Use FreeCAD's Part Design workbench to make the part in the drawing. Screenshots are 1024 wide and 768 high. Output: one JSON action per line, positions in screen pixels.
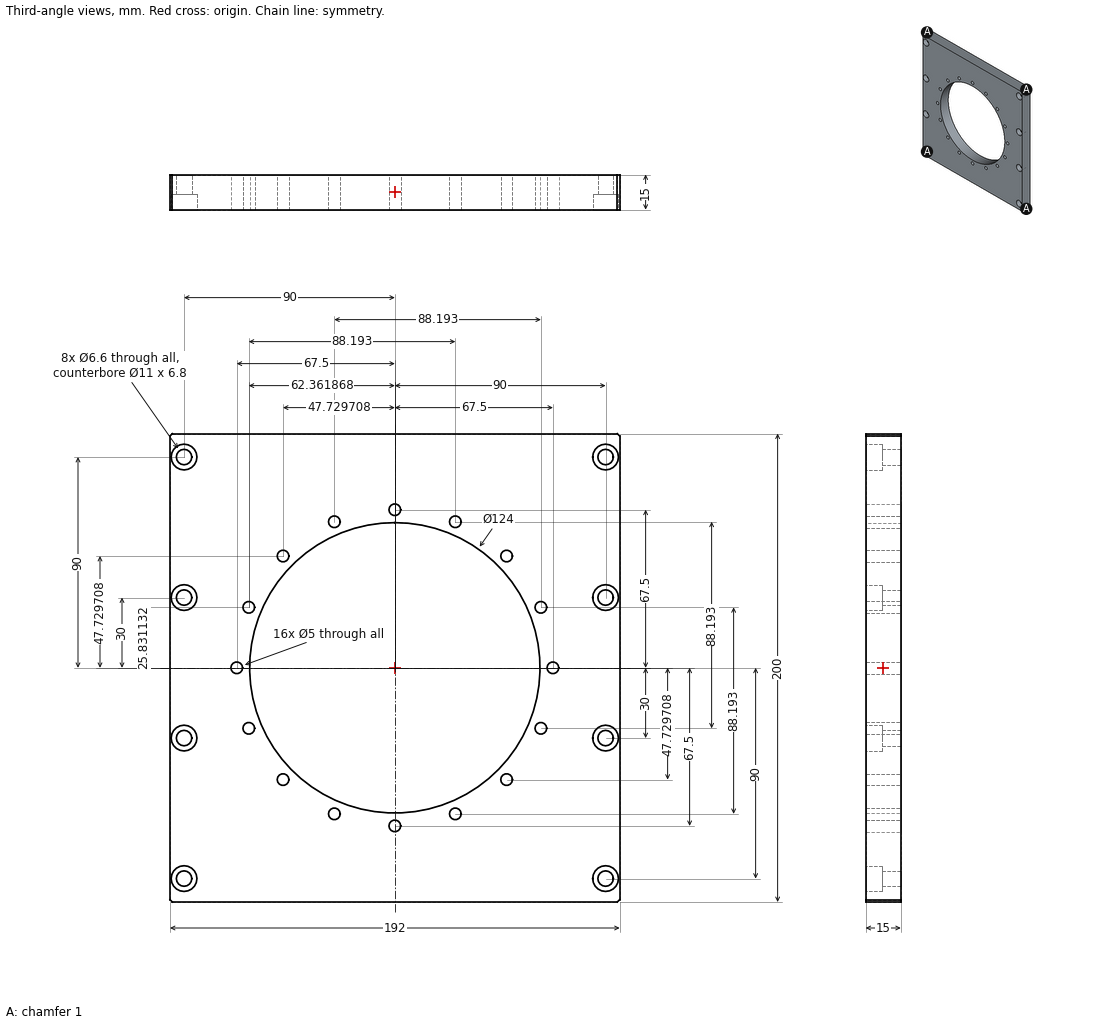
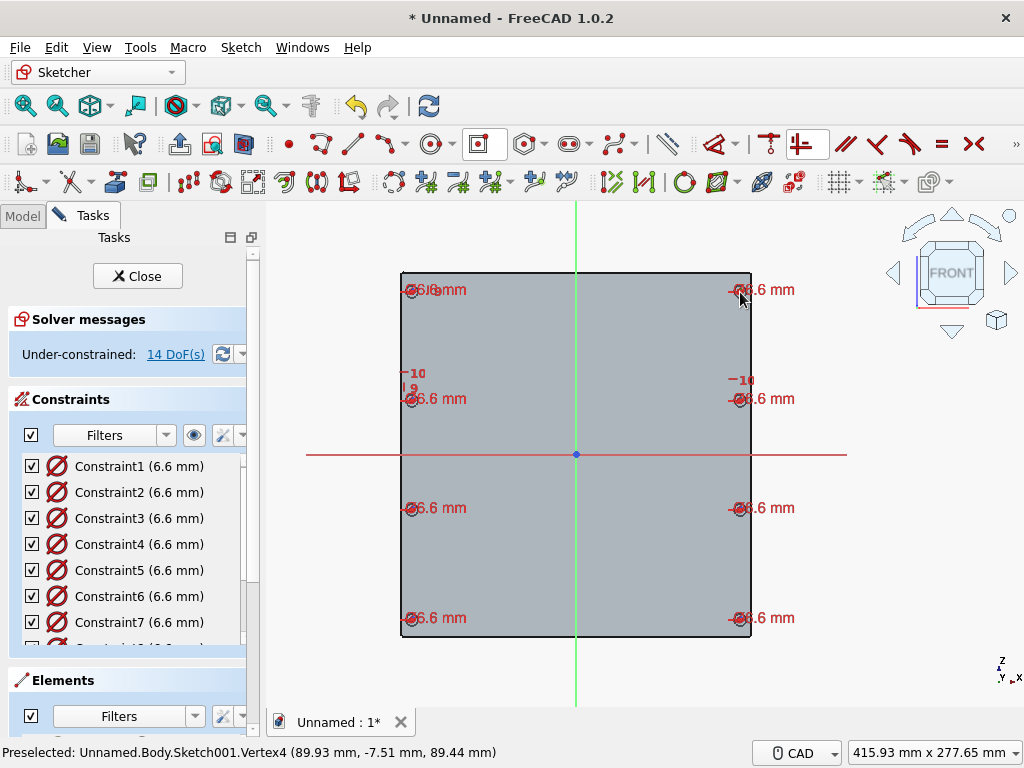
{"action": "left_click", "coordinate": [824, 144]}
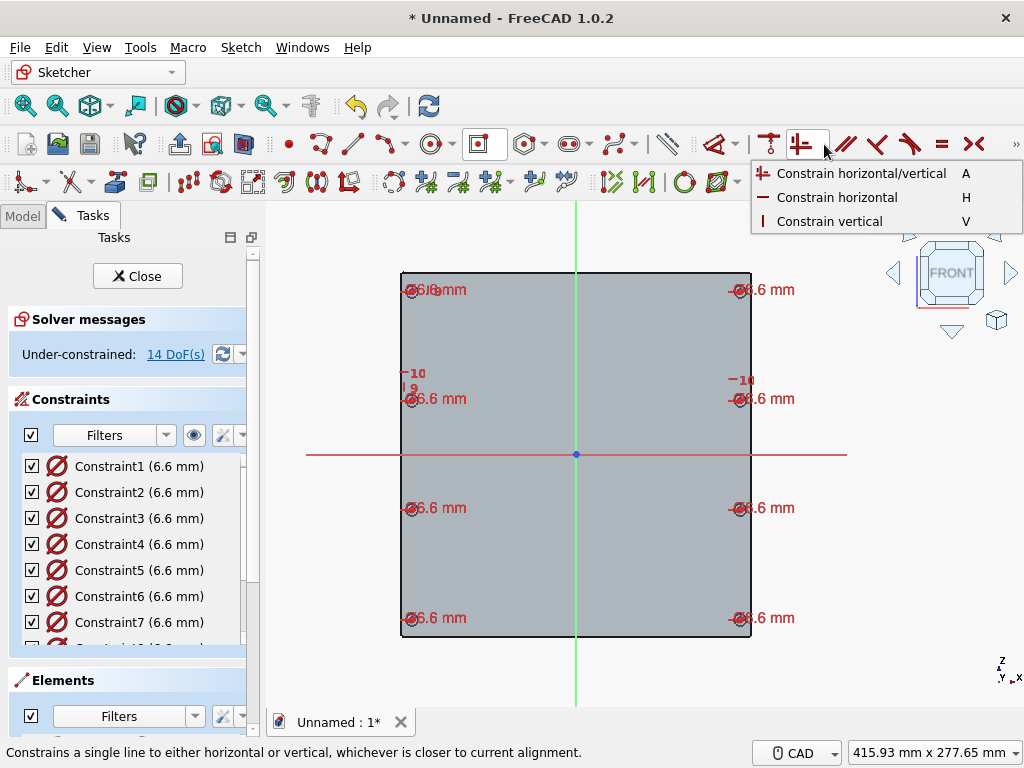
{"action": "left_click", "coordinate": [887, 221]}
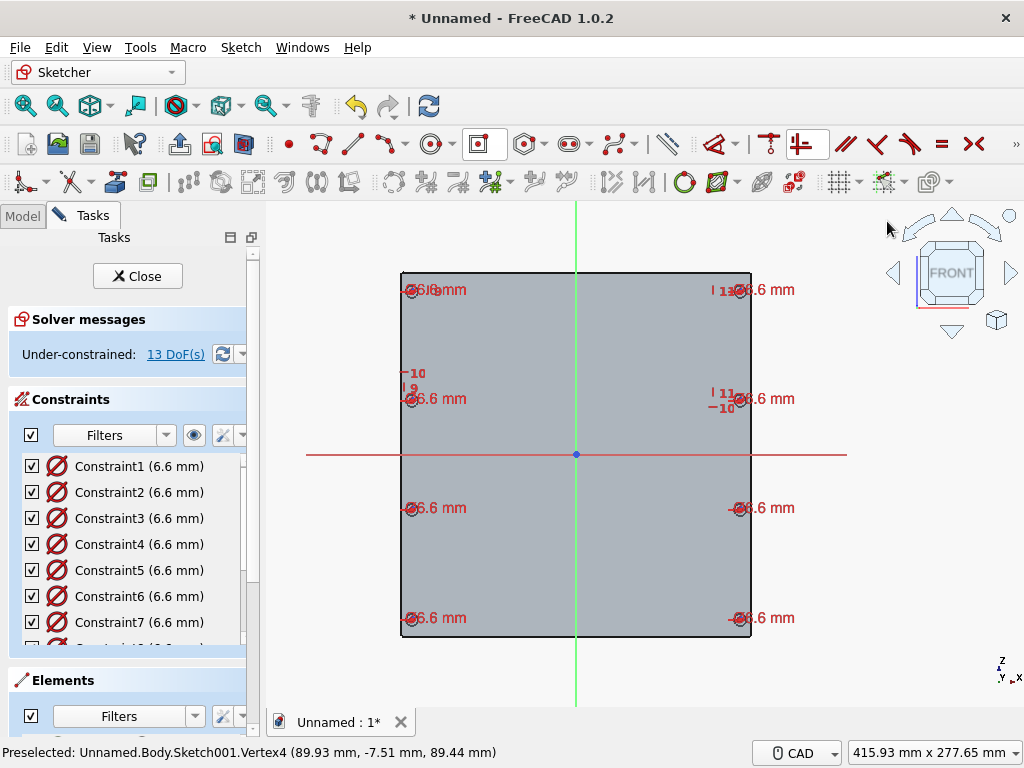
{"action": "left_click", "coordinate": [412, 292]}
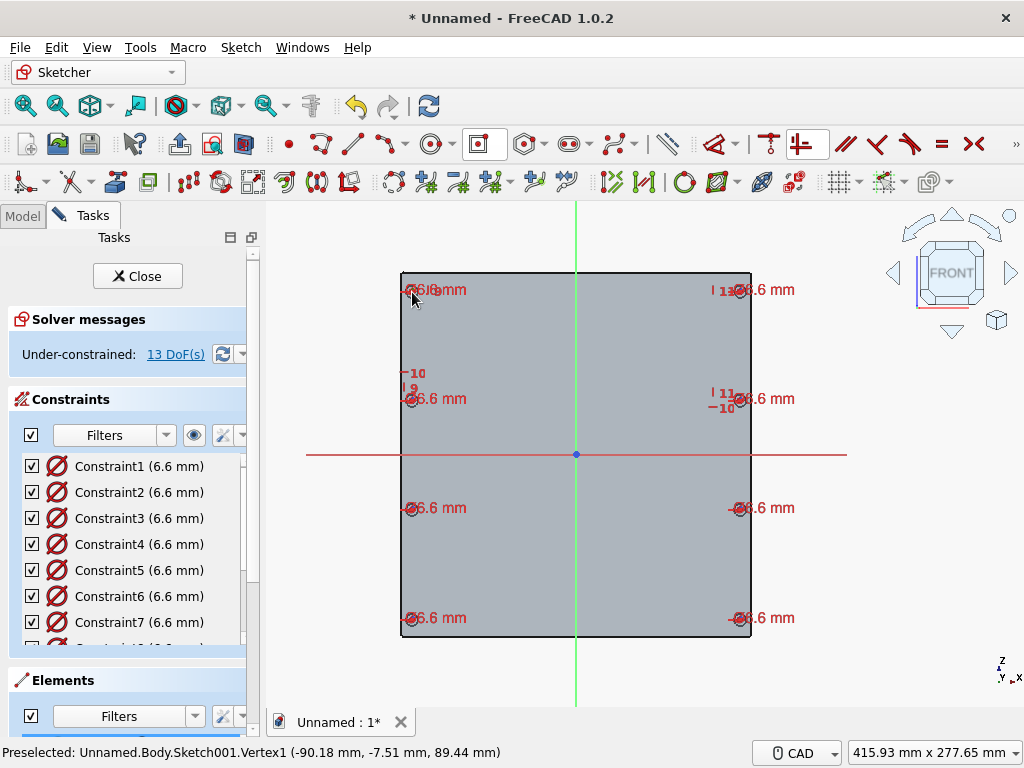
{"action": "left_click", "coordinate": [740, 292]}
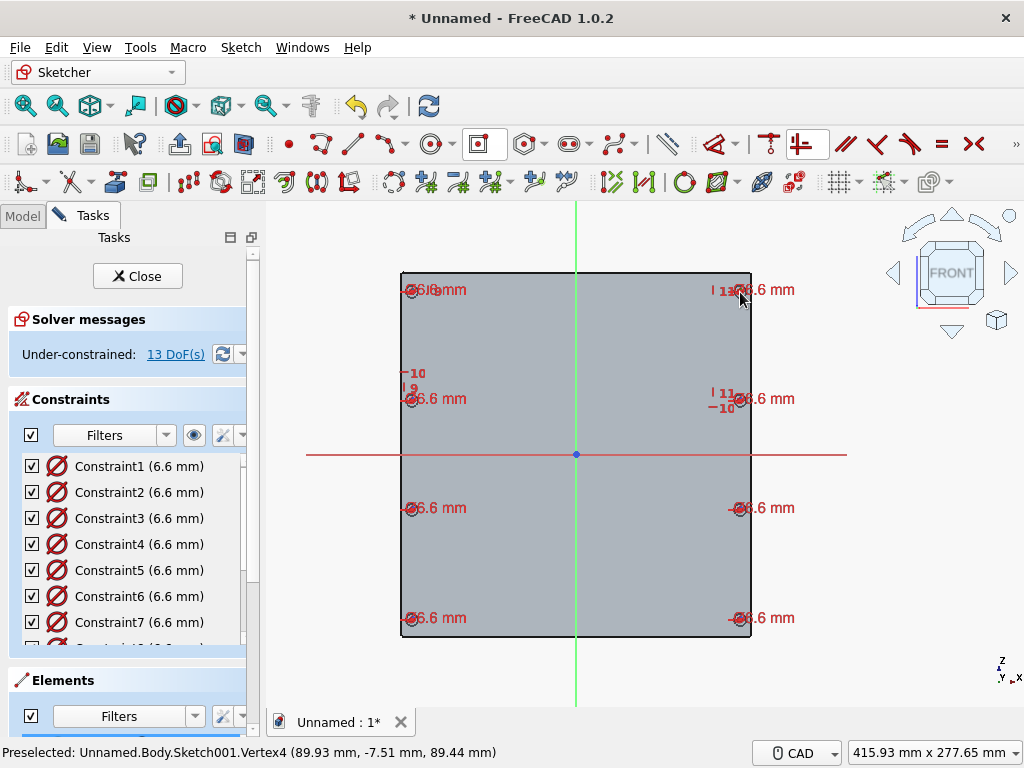
{"action": "left_click", "coordinate": [824, 144]}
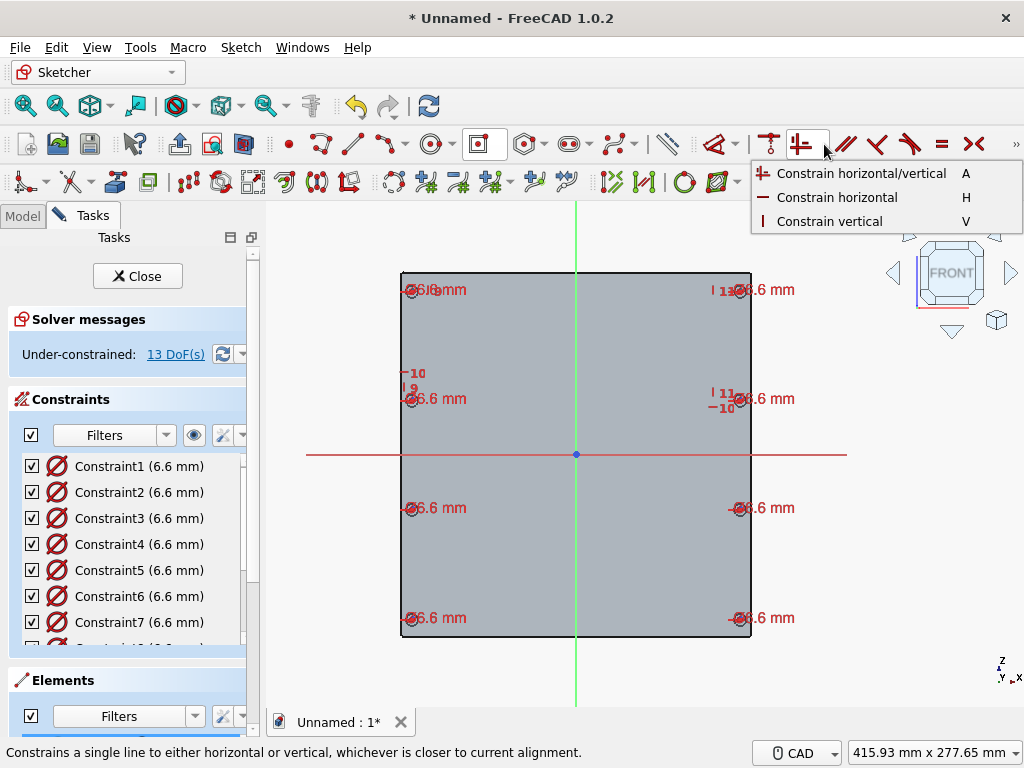
{"action": "left_click", "coordinate": [887, 197]}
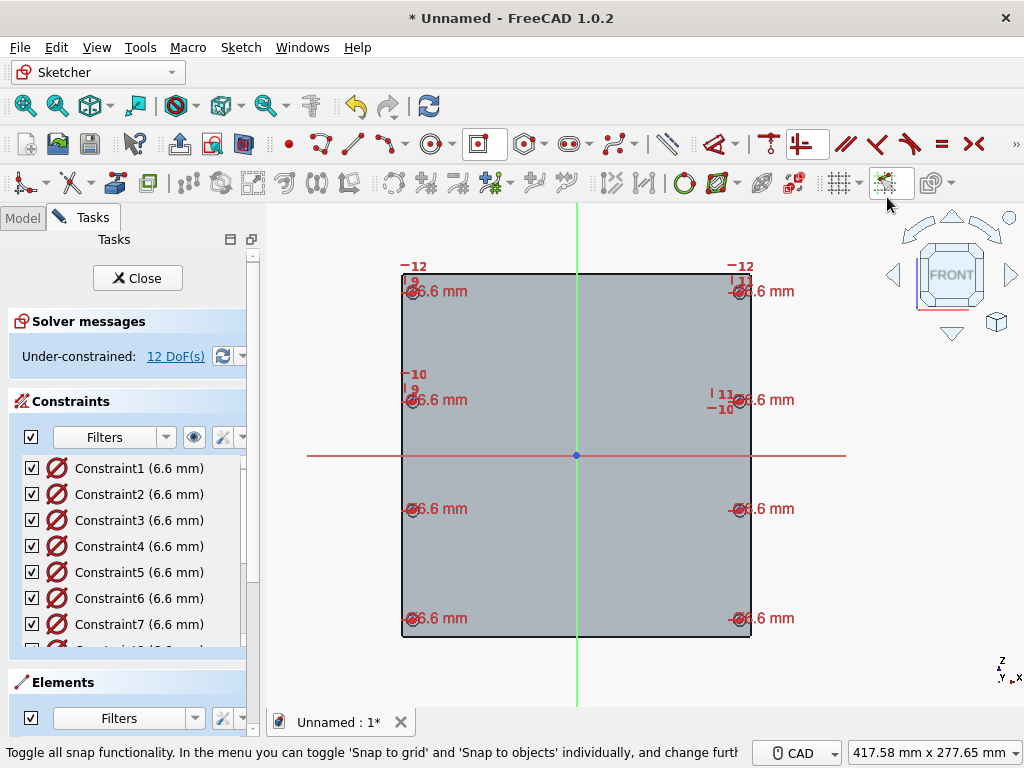
{"action": "left_click", "coordinate": [740, 402]}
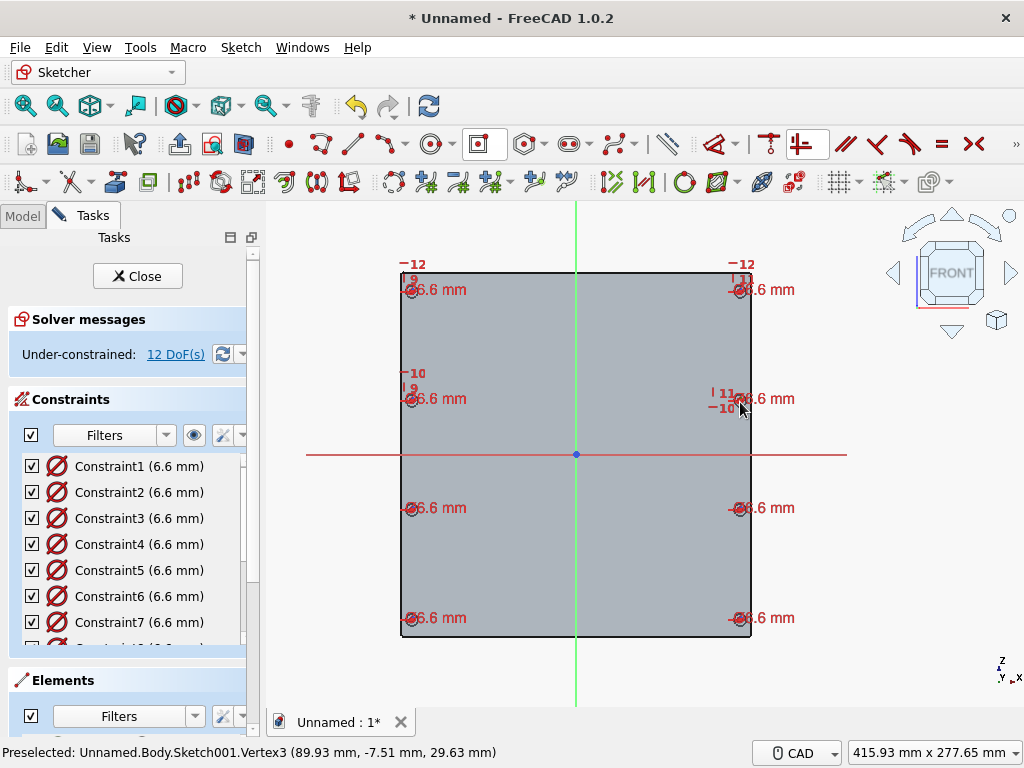
{"action": "left_click", "coordinate": [740, 620]}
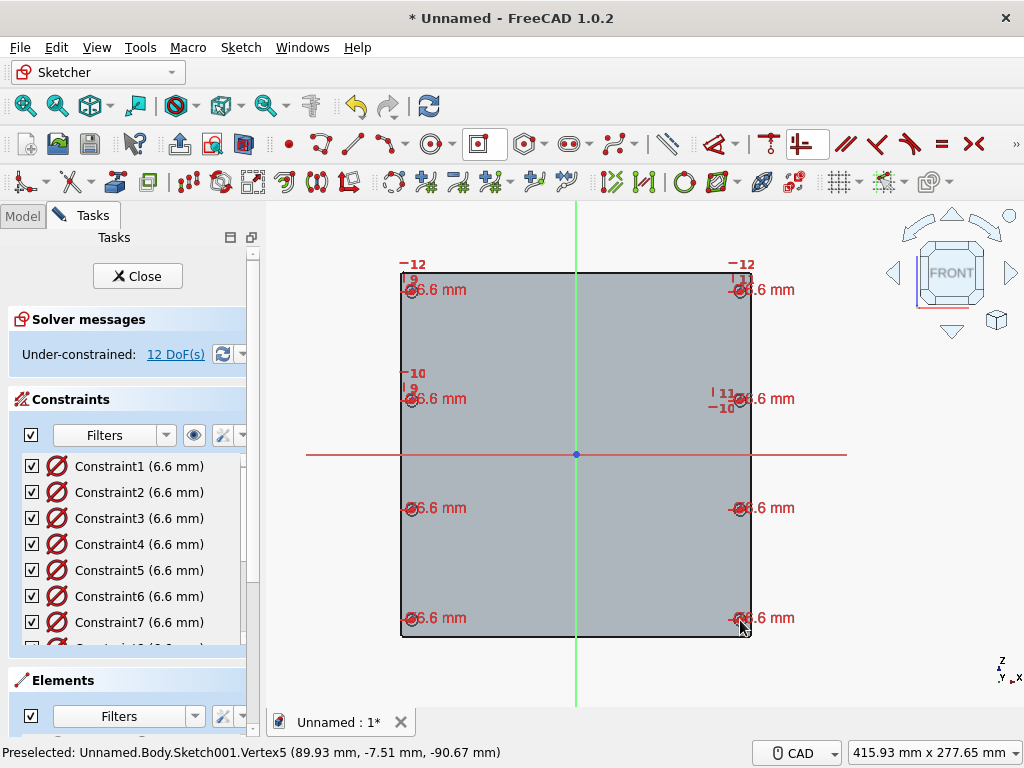
{"action": "key", "text": "v"}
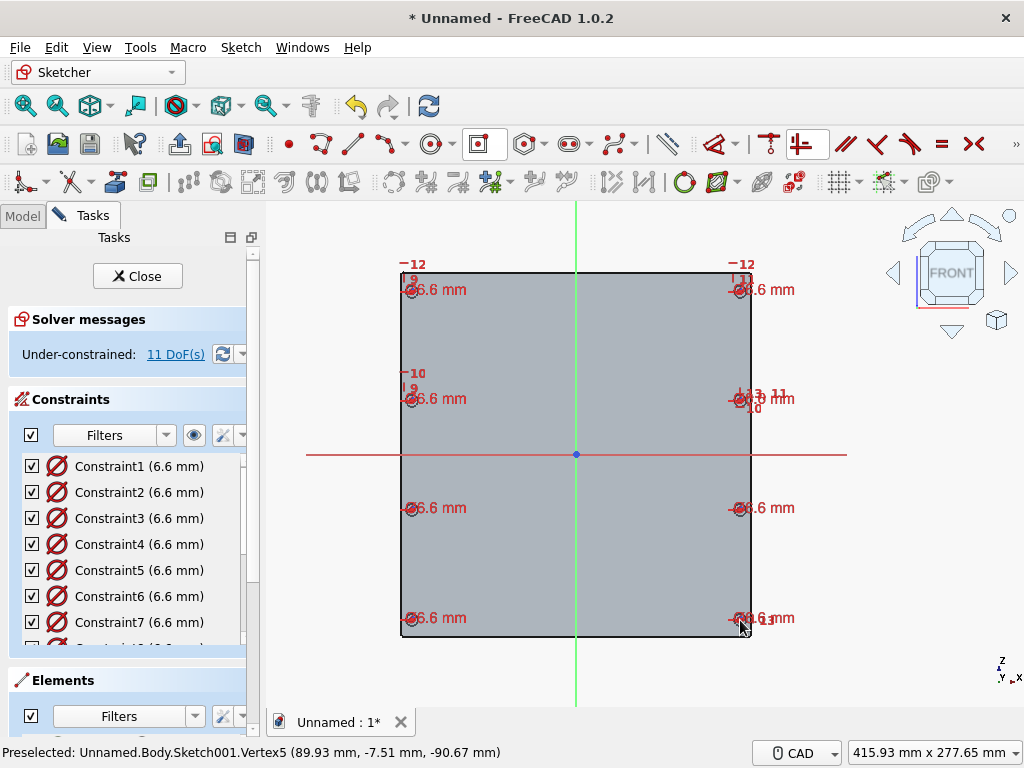
{"action": "left_click", "coordinate": [740, 401]}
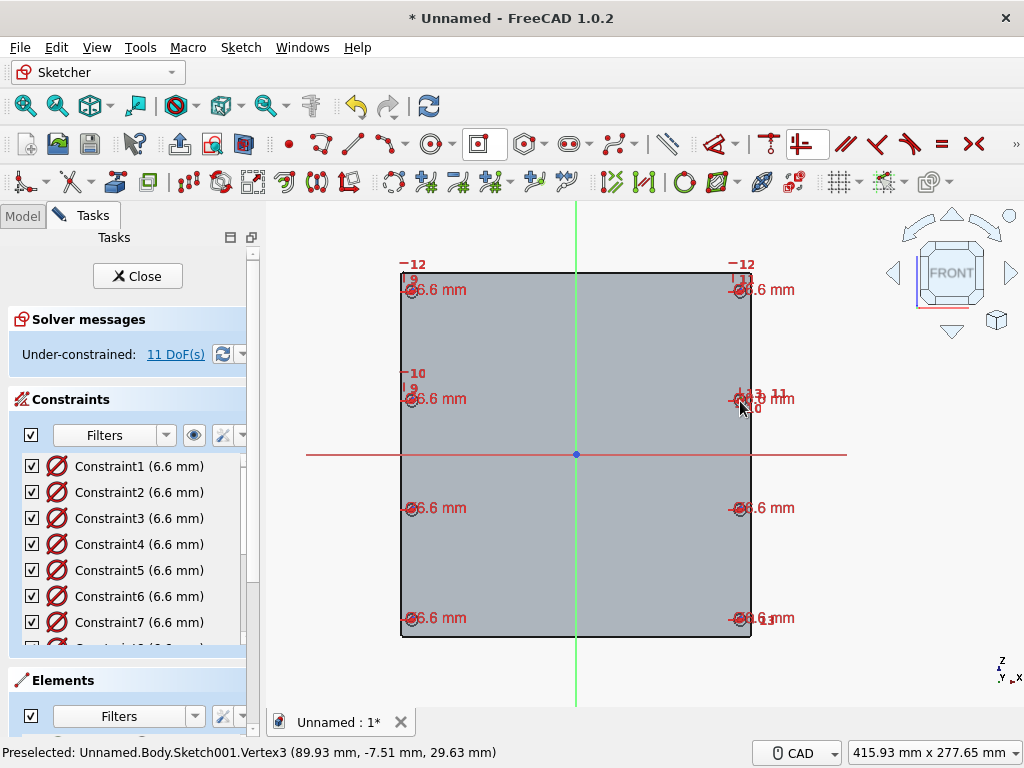
{"action": "left_click", "coordinate": [740, 510]}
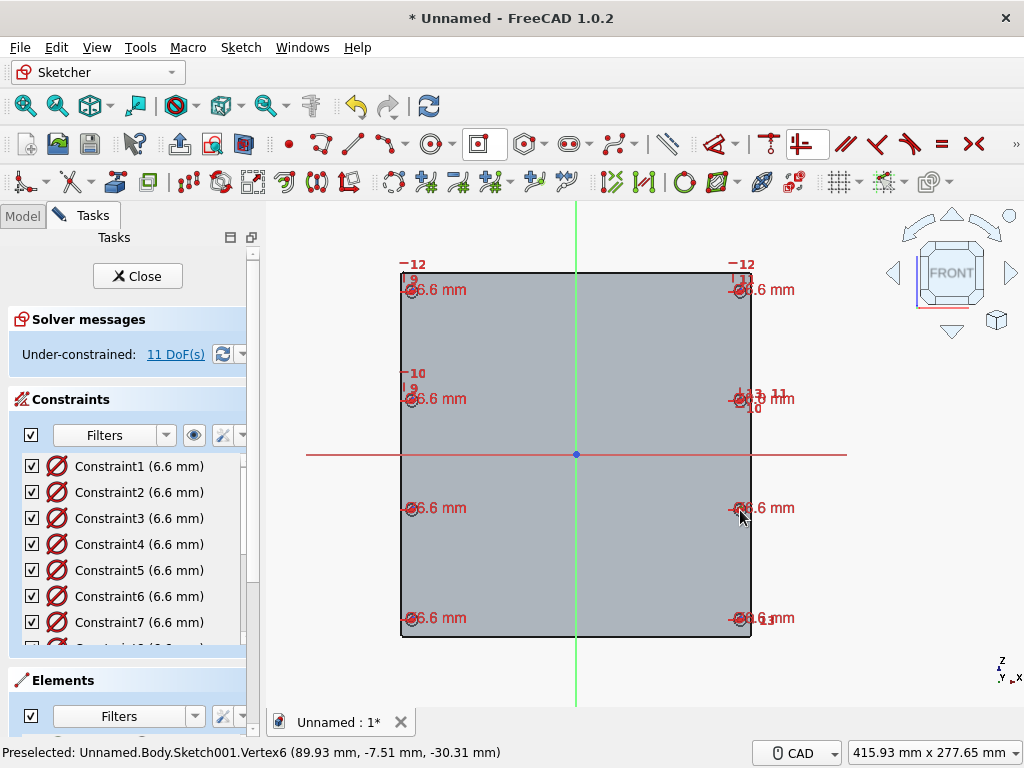
{"action": "key", "text": "v"}